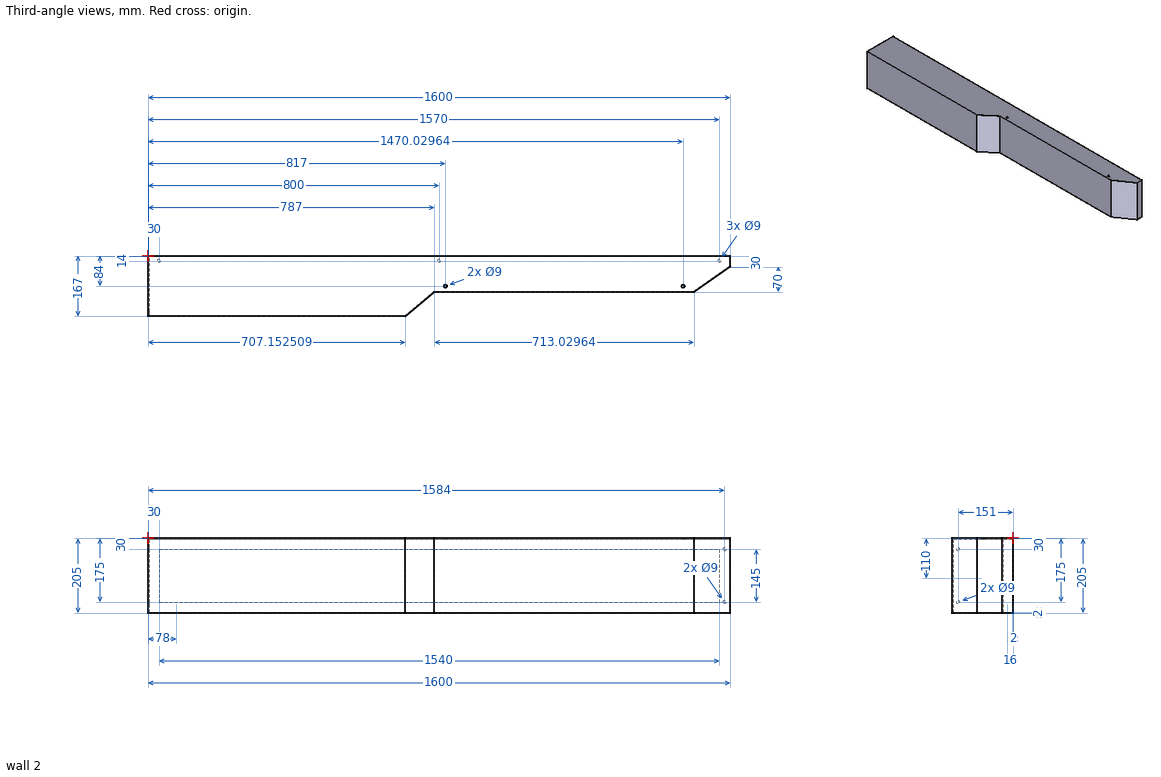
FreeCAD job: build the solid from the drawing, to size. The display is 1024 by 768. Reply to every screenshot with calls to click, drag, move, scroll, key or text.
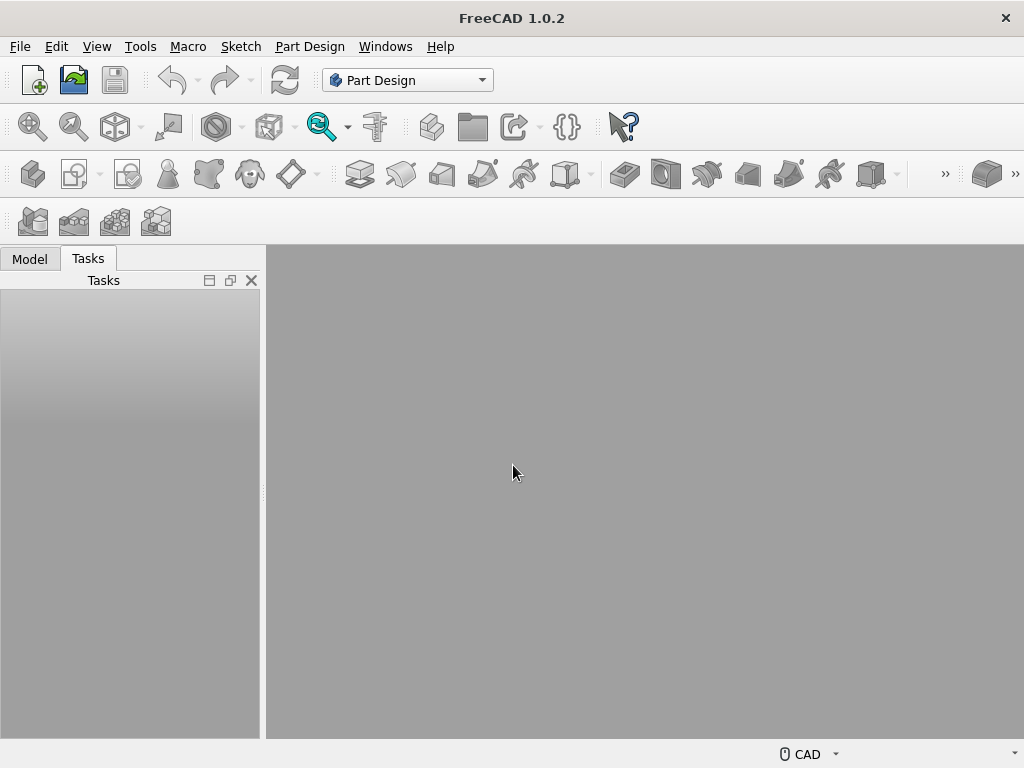
click(33, 80)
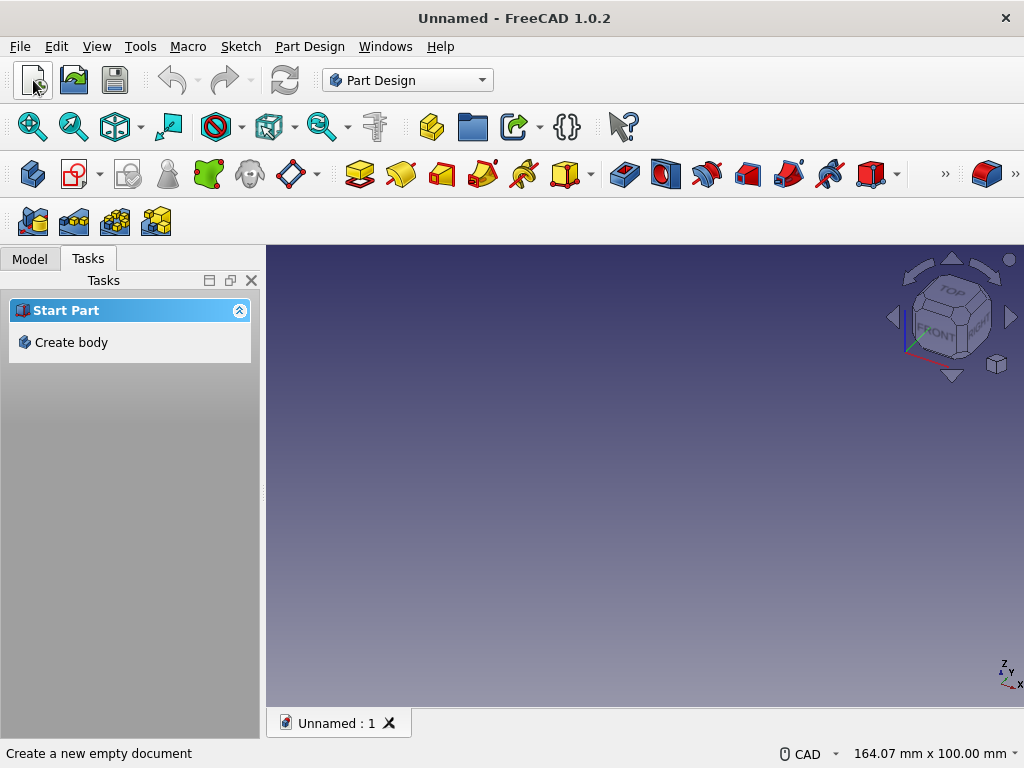
click(74, 174)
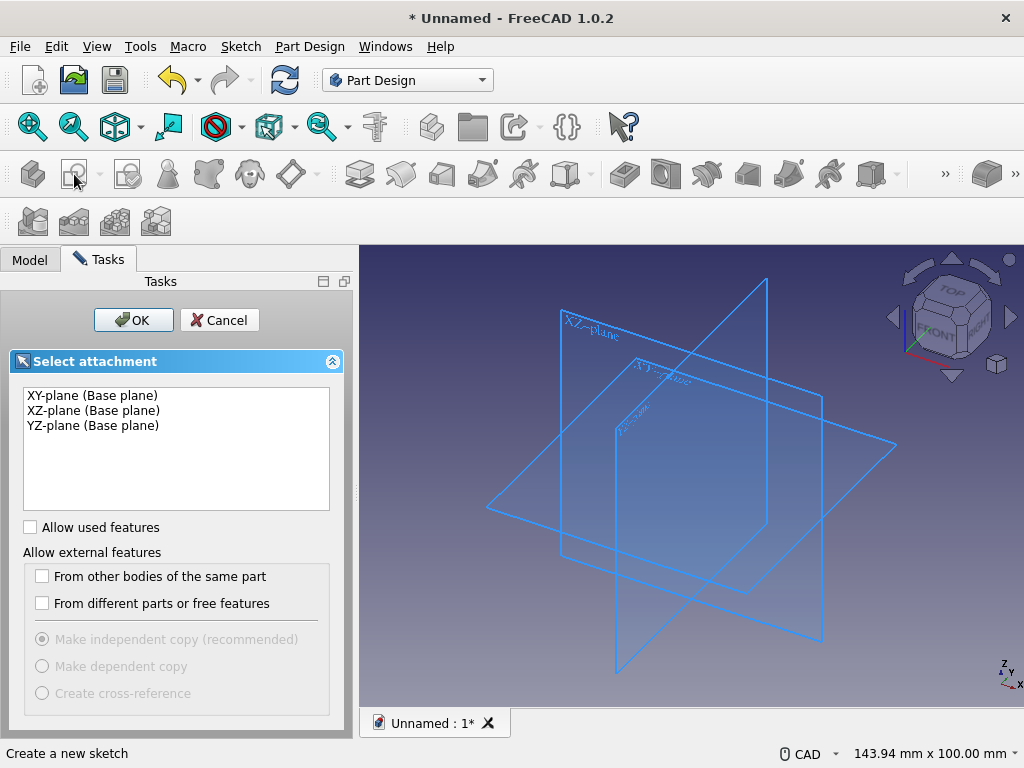
click(84, 396)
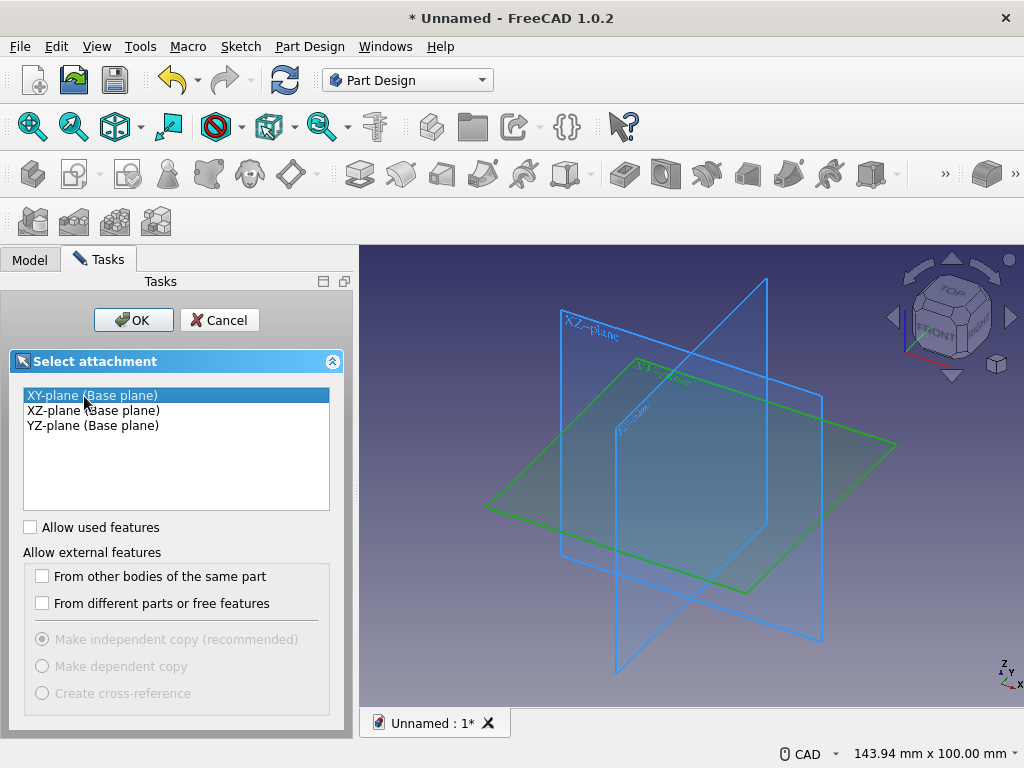
click(134, 320)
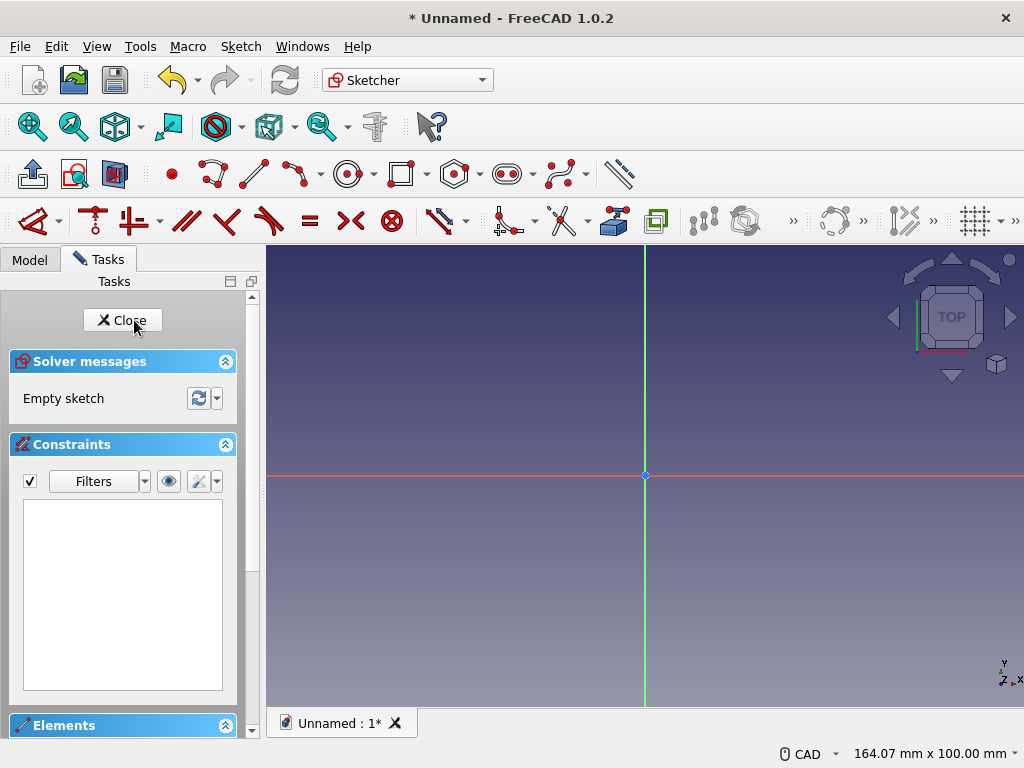
scroll(379, 456, down, 15)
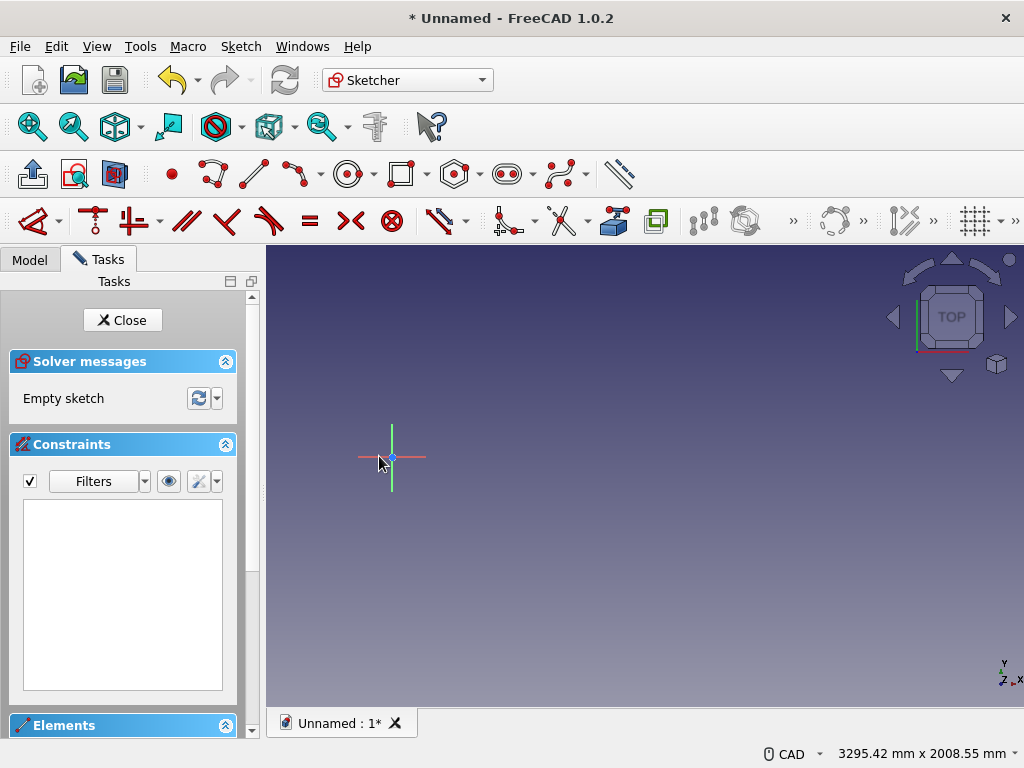
key(g)
key(m)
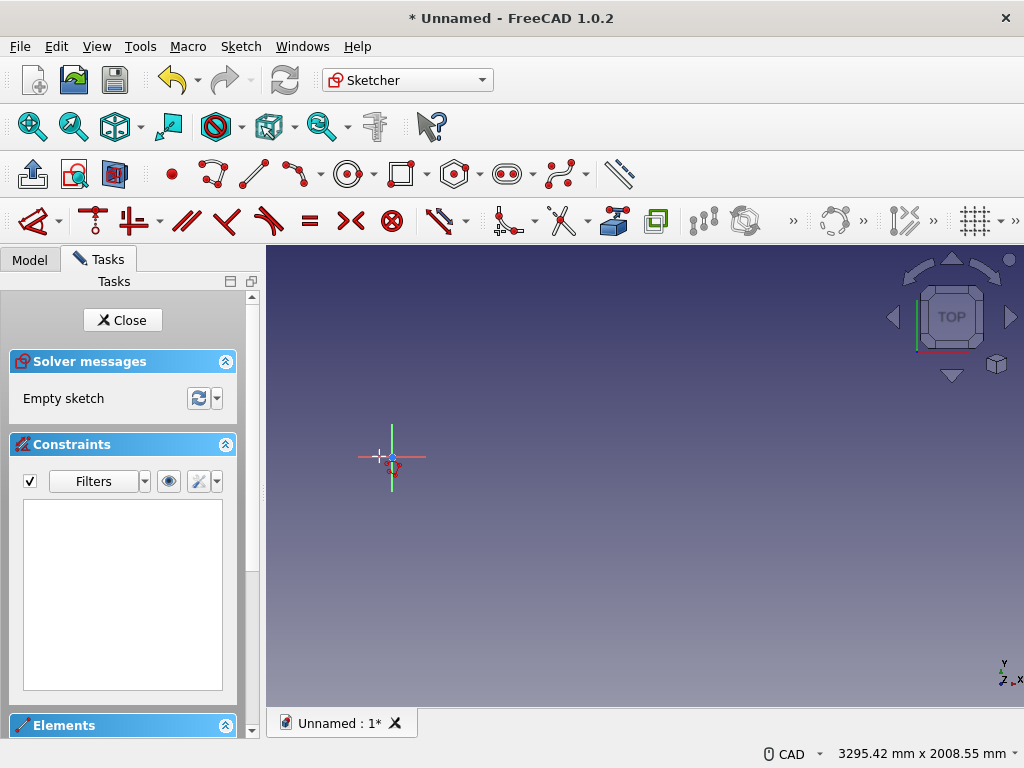
click(392, 457)
click(760, 466)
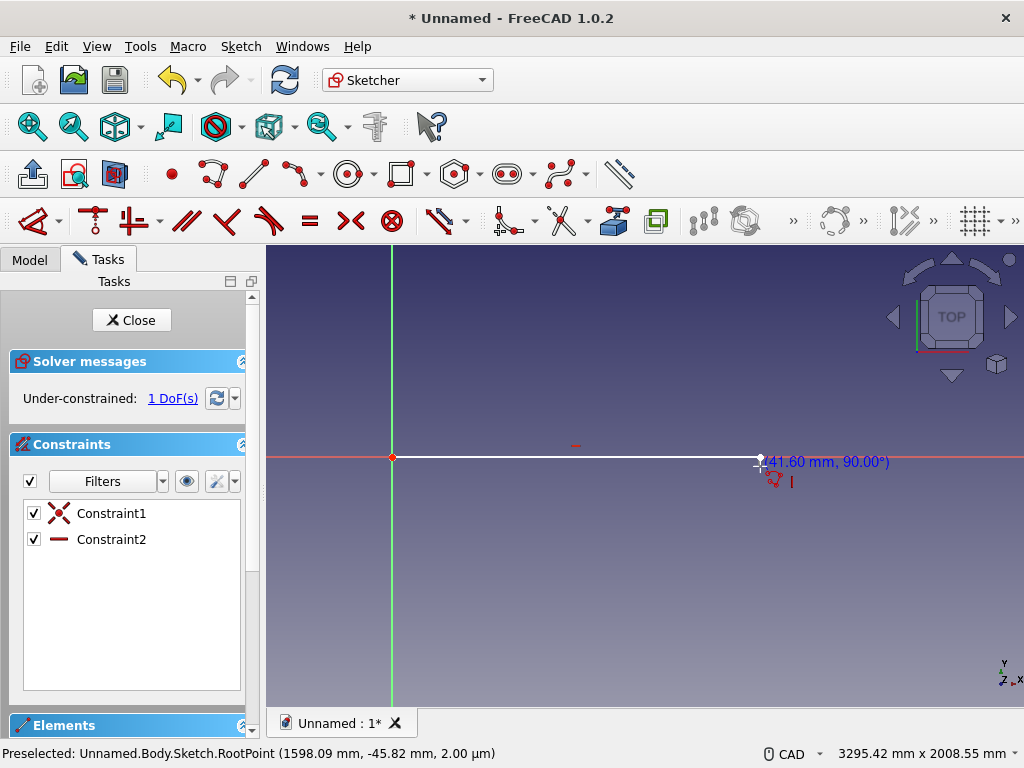
scroll(760, 464, up, 5)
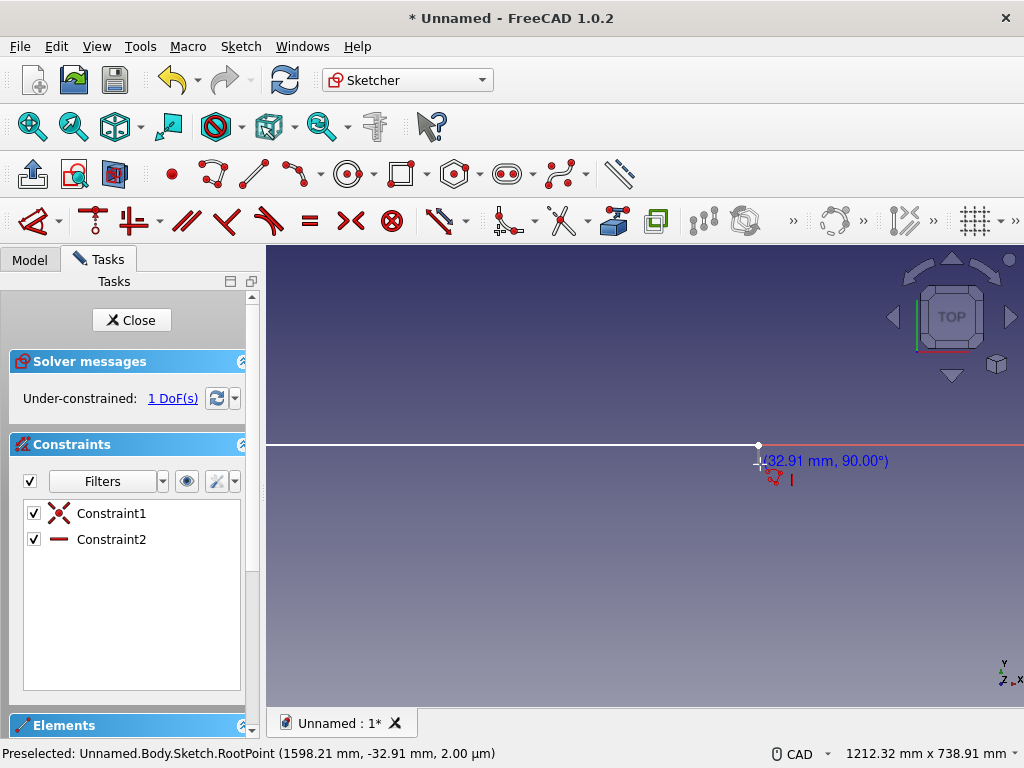
click(759, 464)
click(697, 508)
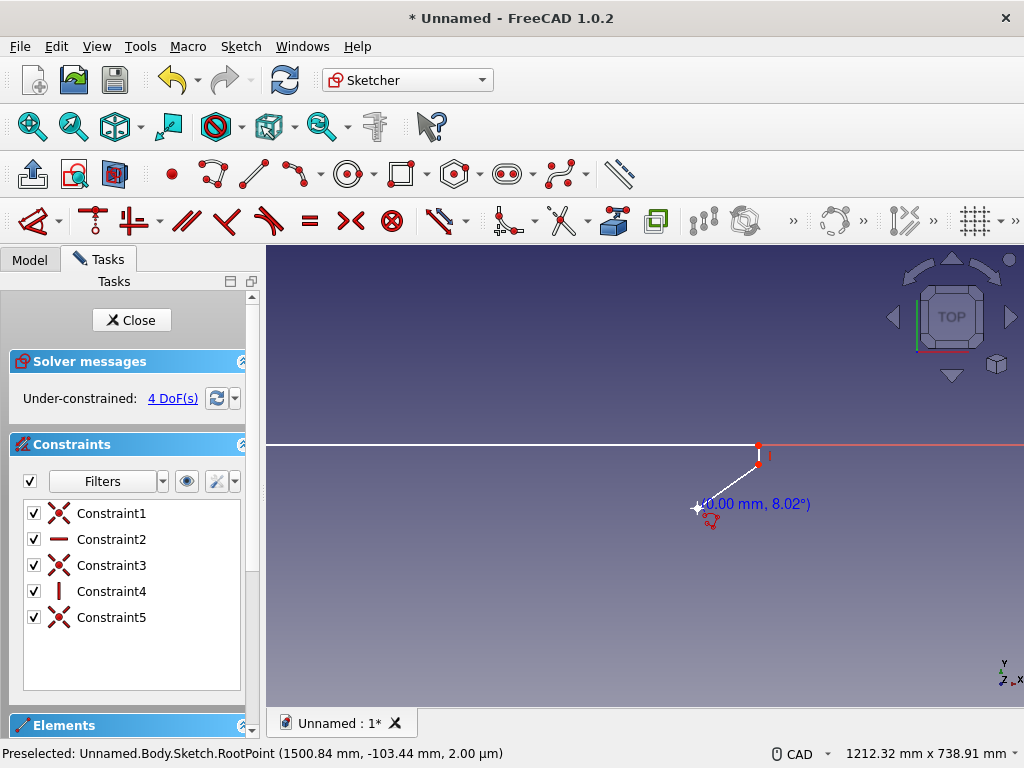
scroll(761, 463, down, 5)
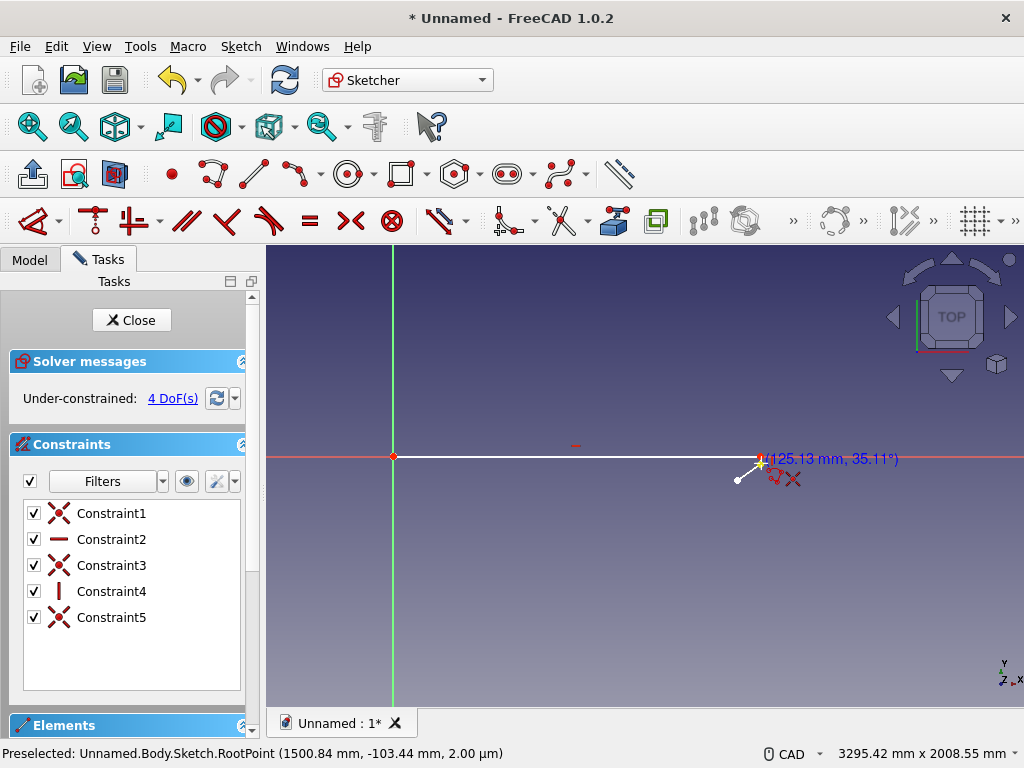
click(574, 480)
click(556, 495)
click(402, 495)
click(393, 457)
key(Escape)
key(Escape)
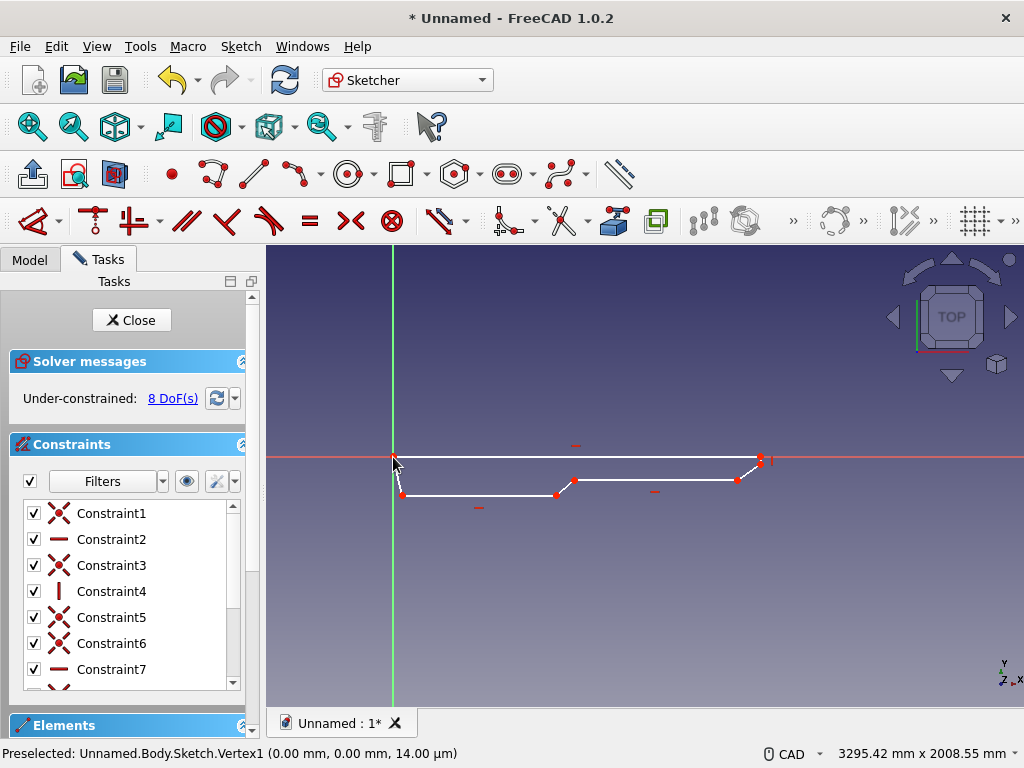
click(396, 469)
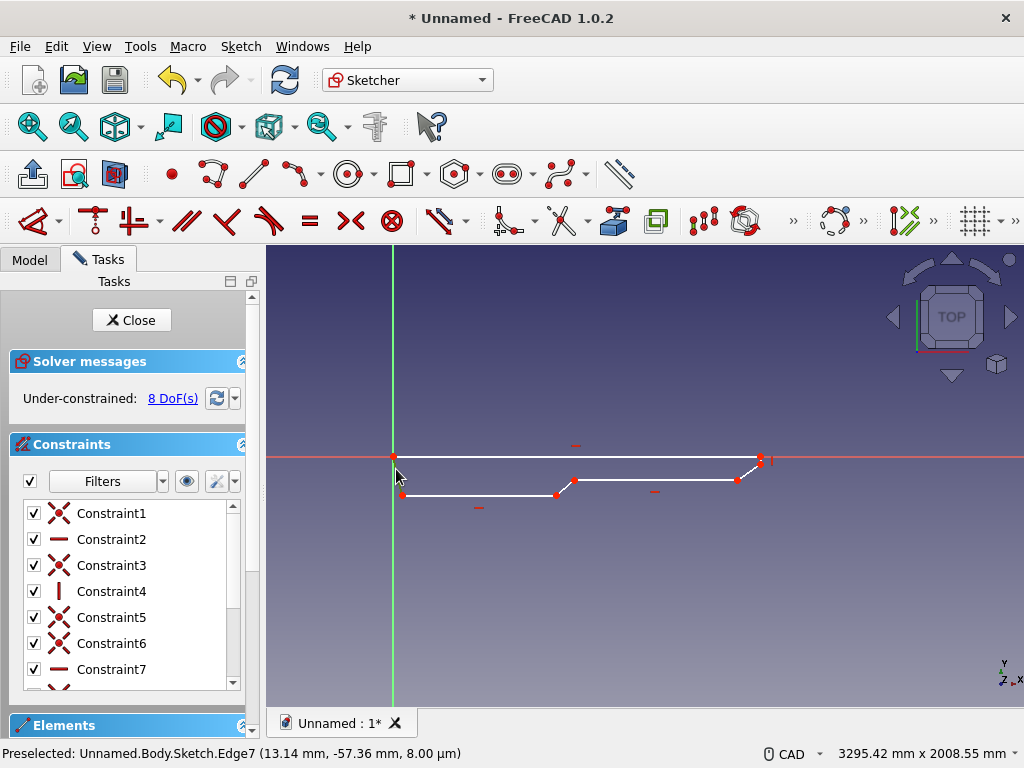
click(160, 222)